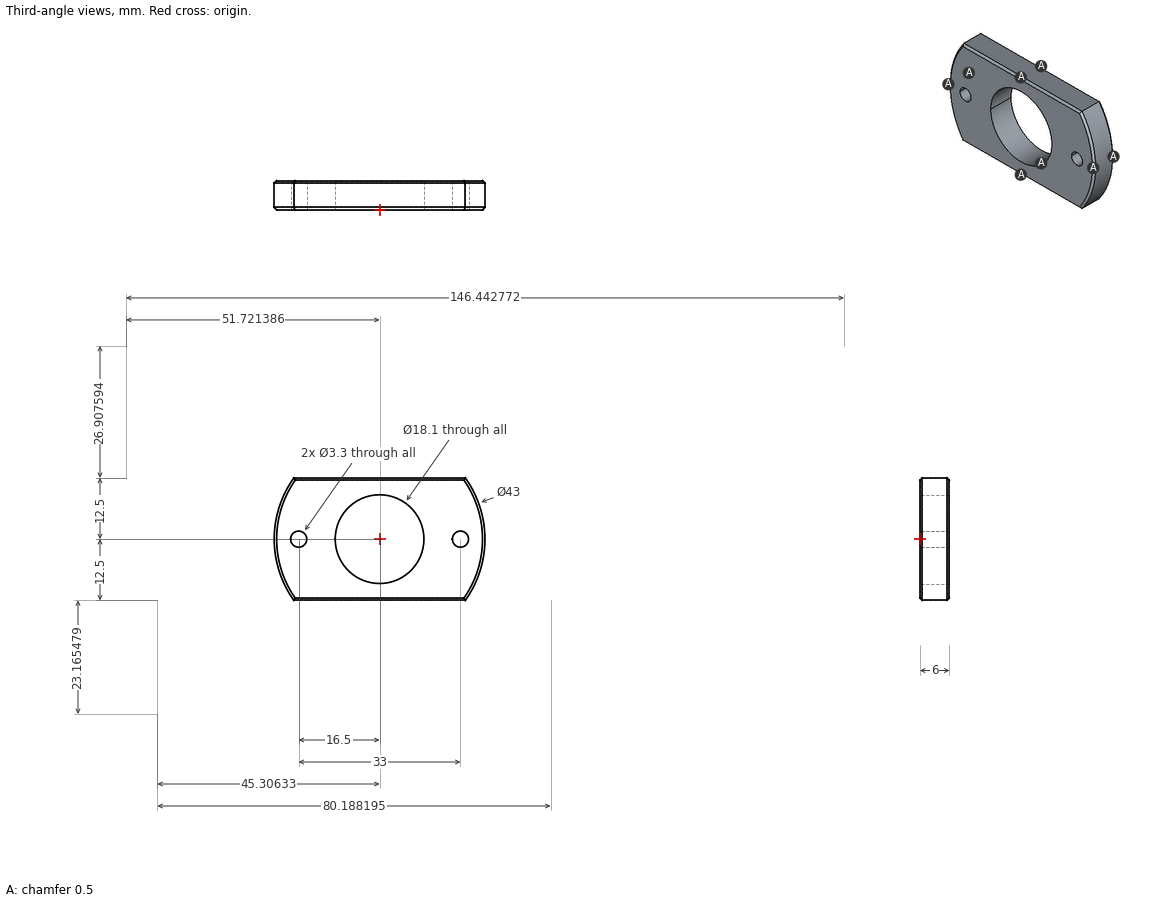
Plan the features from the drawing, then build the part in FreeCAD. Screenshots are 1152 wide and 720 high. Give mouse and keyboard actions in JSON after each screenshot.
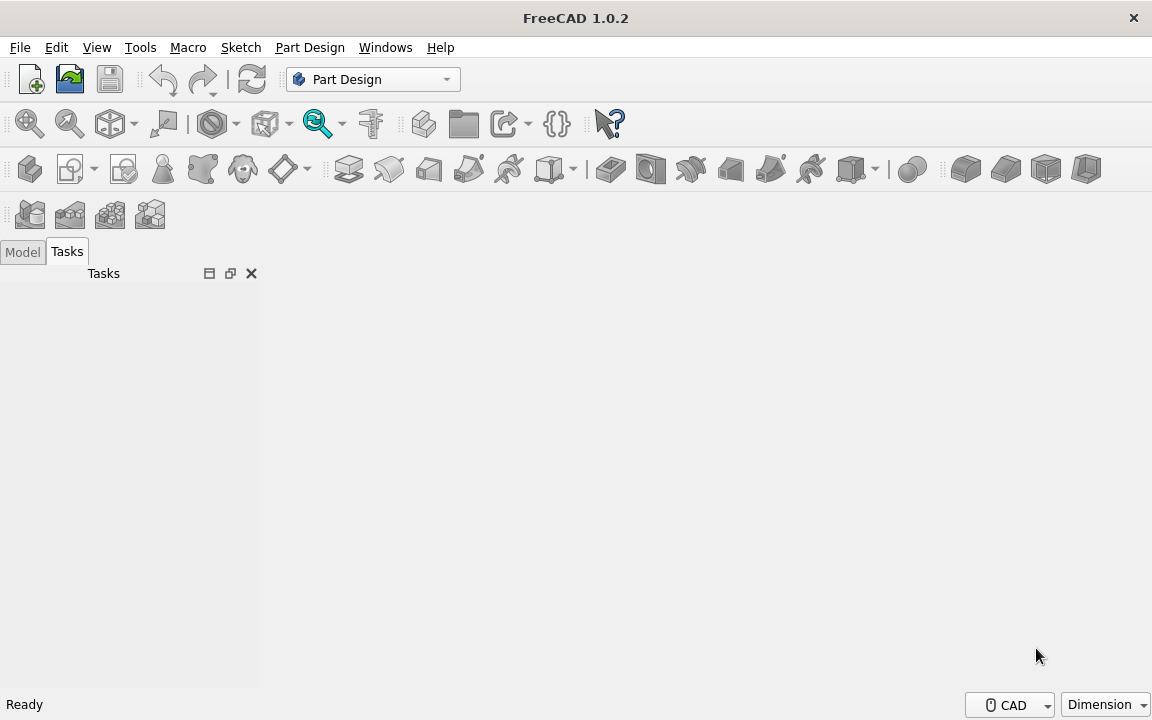
{"action": "left_click", "coordinate": [30, 80]}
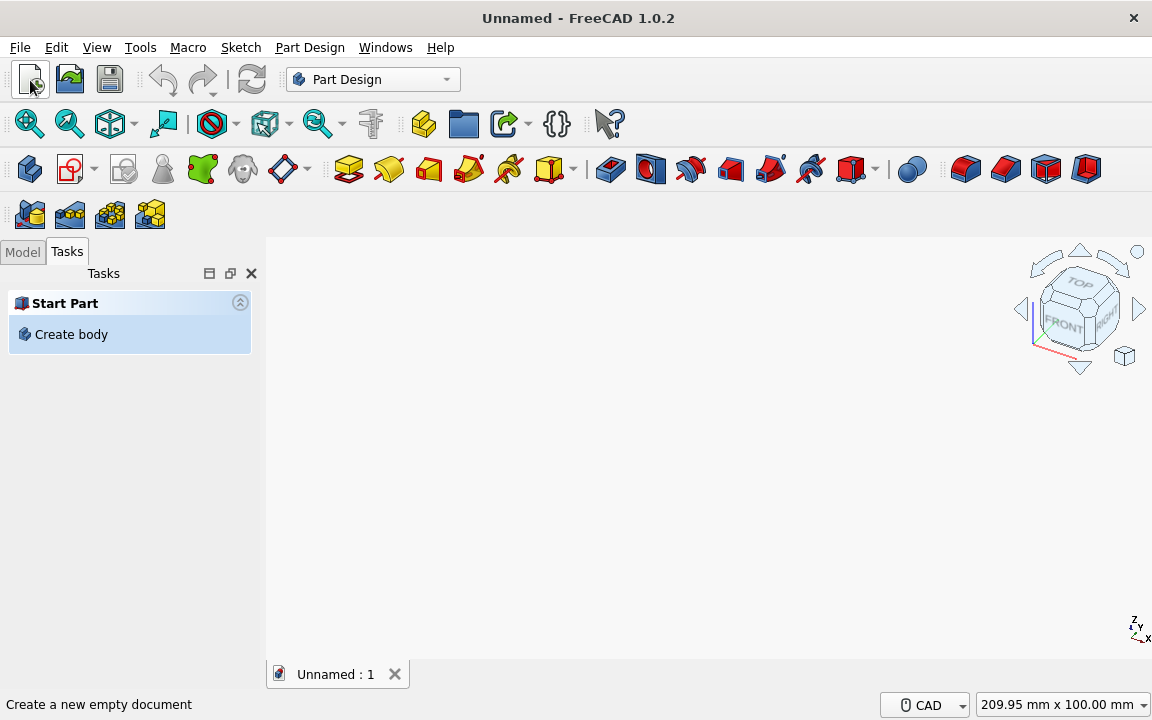
{"action": "left_click", "coordinate": [70, 170]}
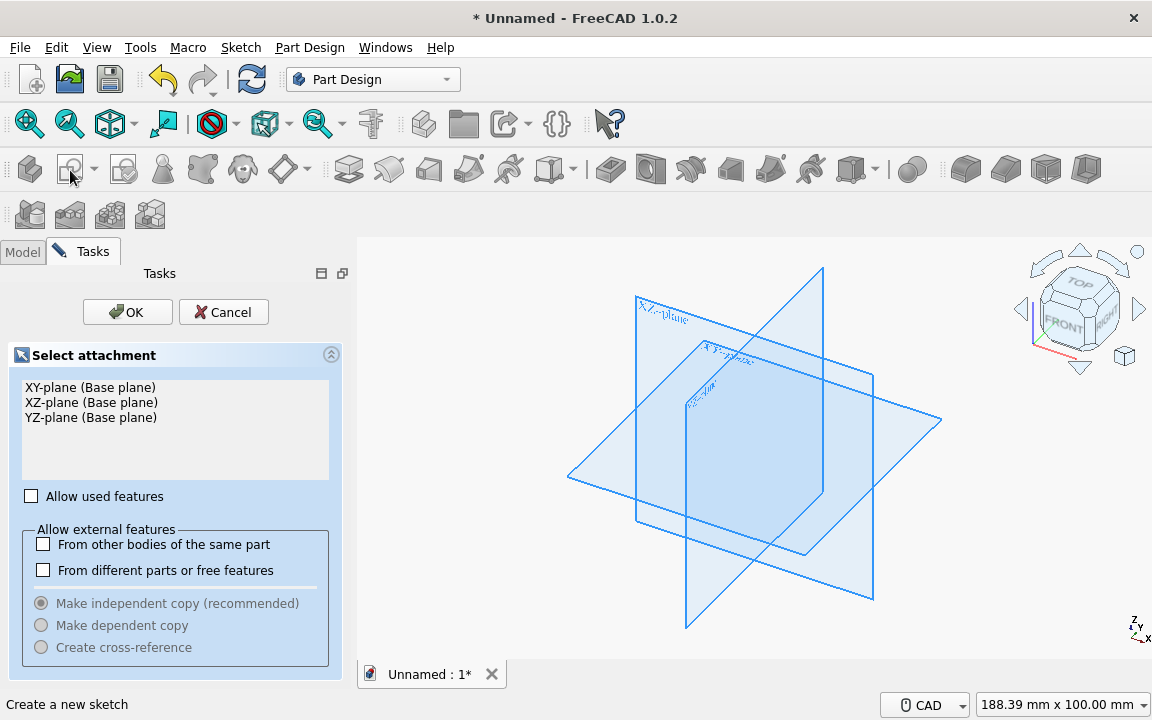
{"action": "left_click", "coordinate": [82, 402]}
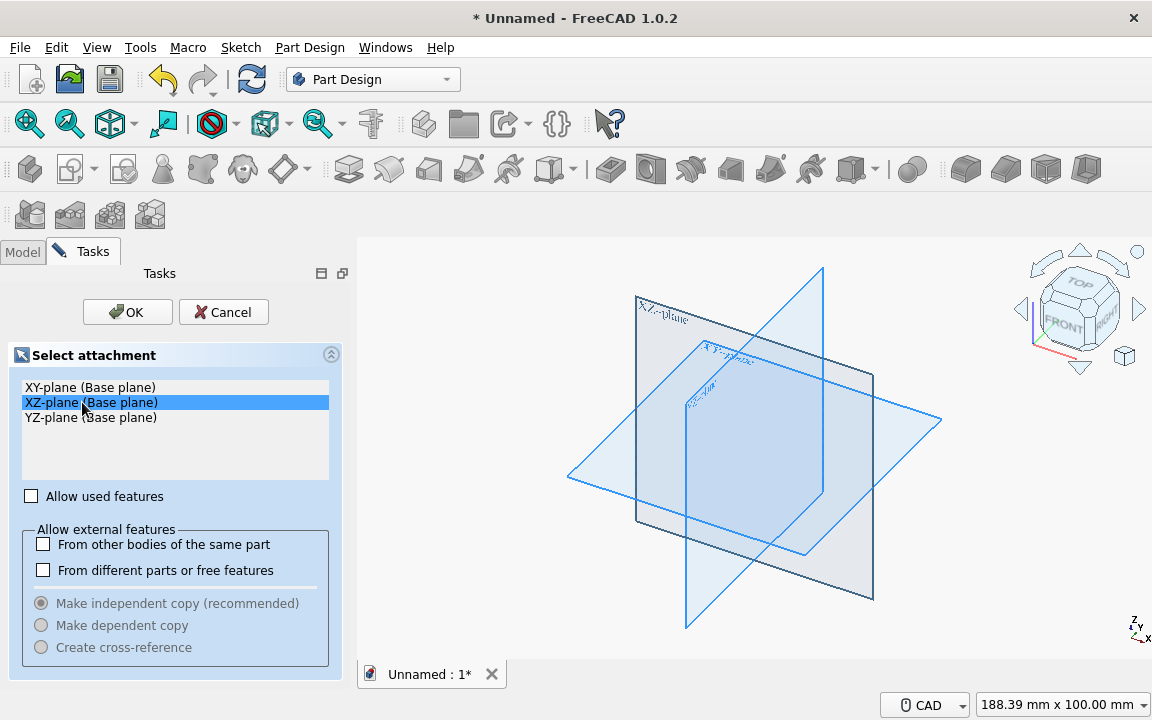
{"action": "left_click", "coordinate": [128, 312]}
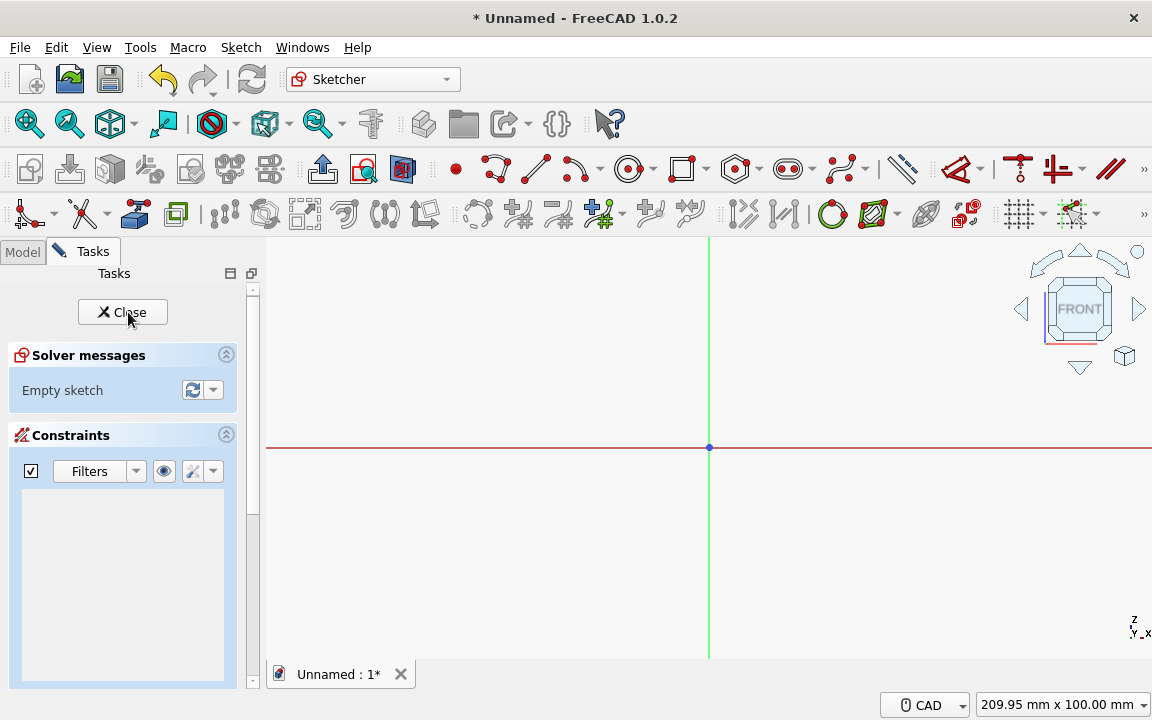
{"action": "scroll", "coordinate": [848, 448], "scroll_direction": "up", "scroll_amount": 2}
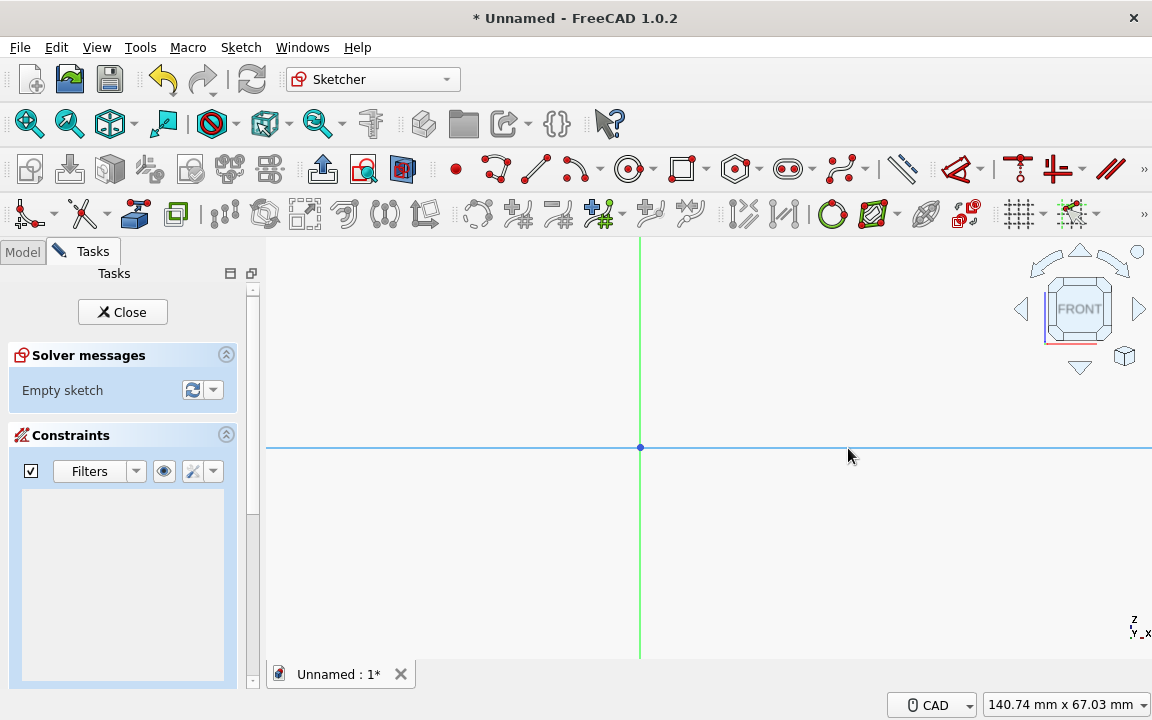
{"action": "left_click", "coordinate": [630, 170]}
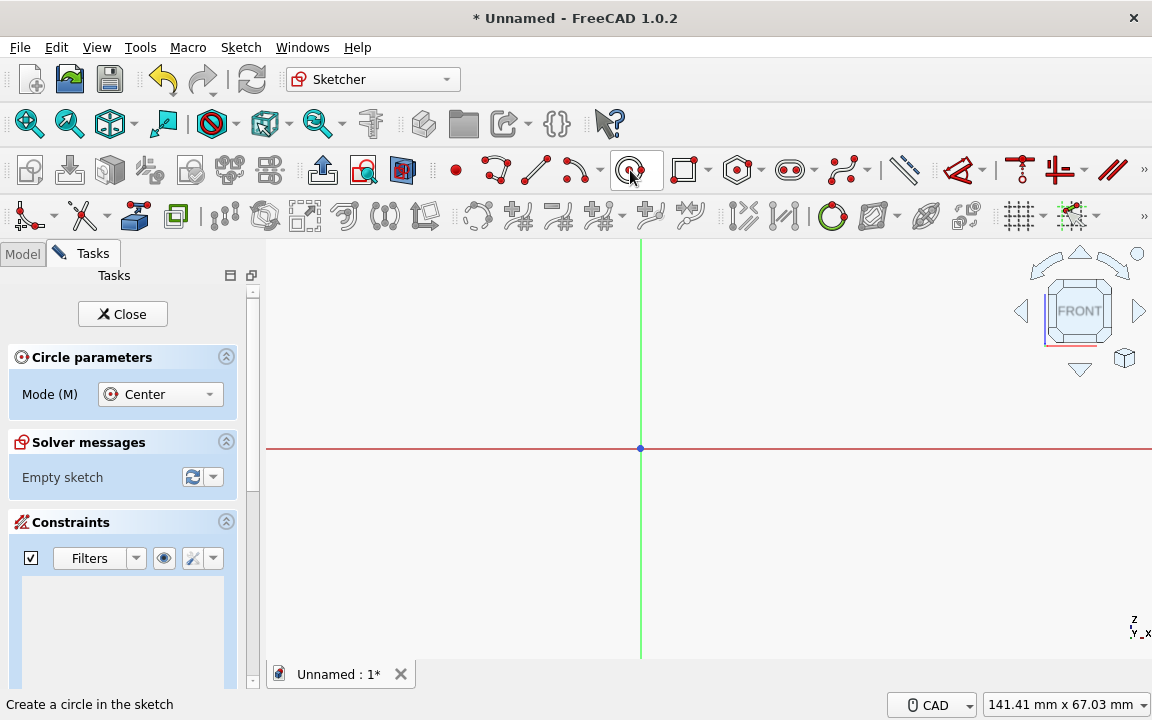
{"action": "left_click", "coordinate": [641, 449]}
{"action": "left_click", "coordinate": [736, 353]}
{"action": "key", "text": "Escape"}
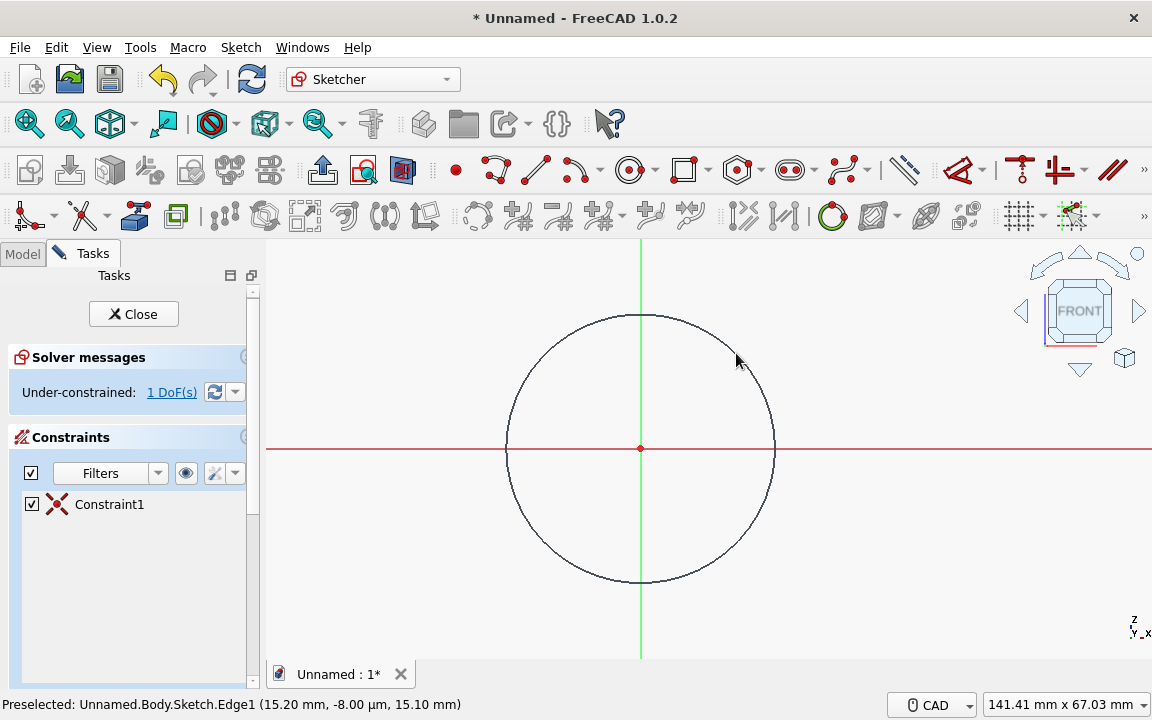
{"action": "left_click", "coordinate": [958, 170]}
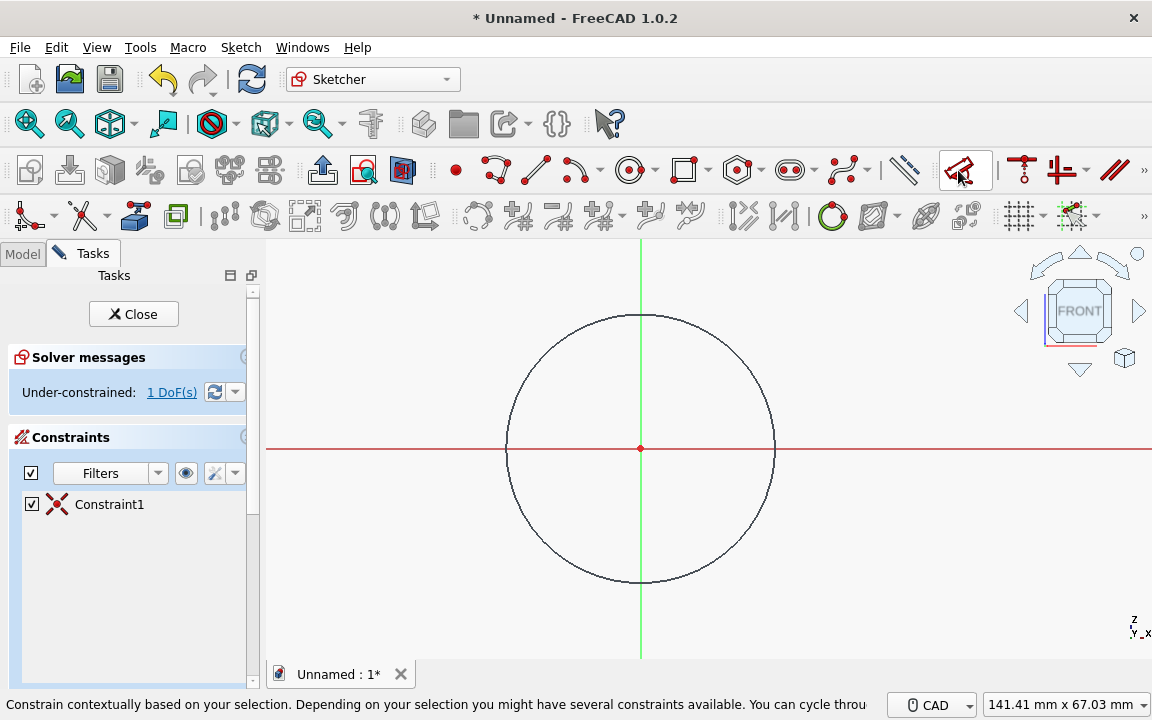
{"action": "left_click", "coordinate": [735, 353]}
{"action": "left_click", "coordinate": [757, 330]}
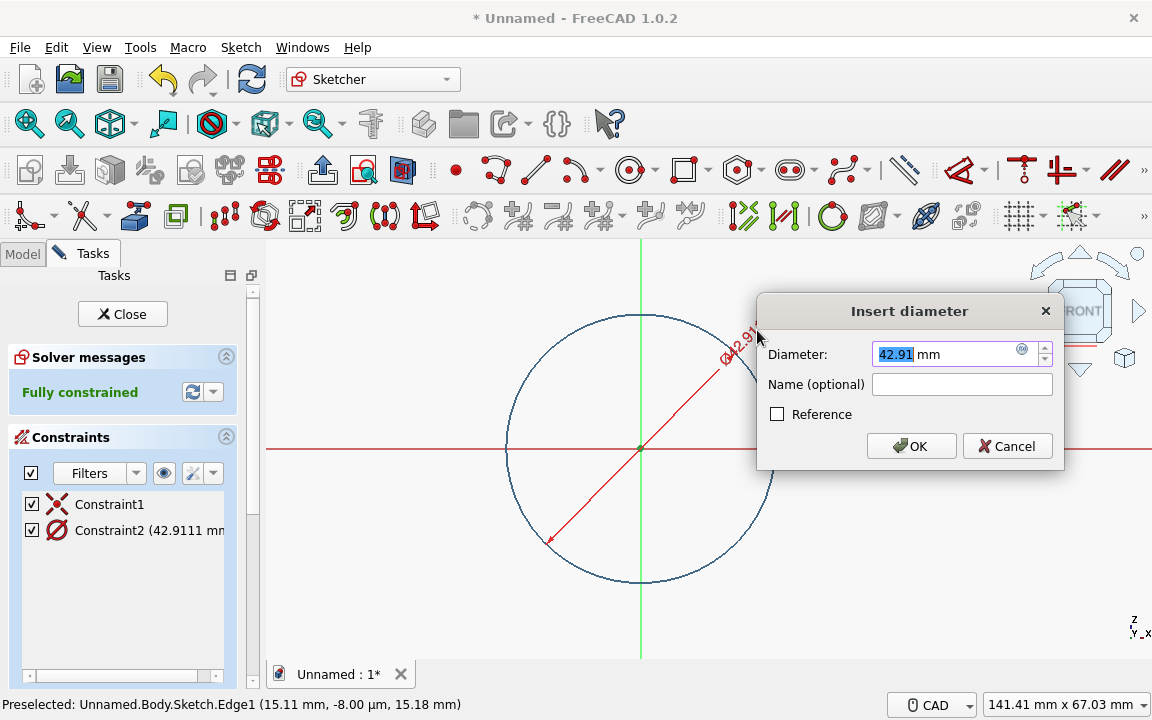
{"action": "type", "text": "43"}
{"action": "key", "text": "Return"}
{"action": "key", "text": "Escape"}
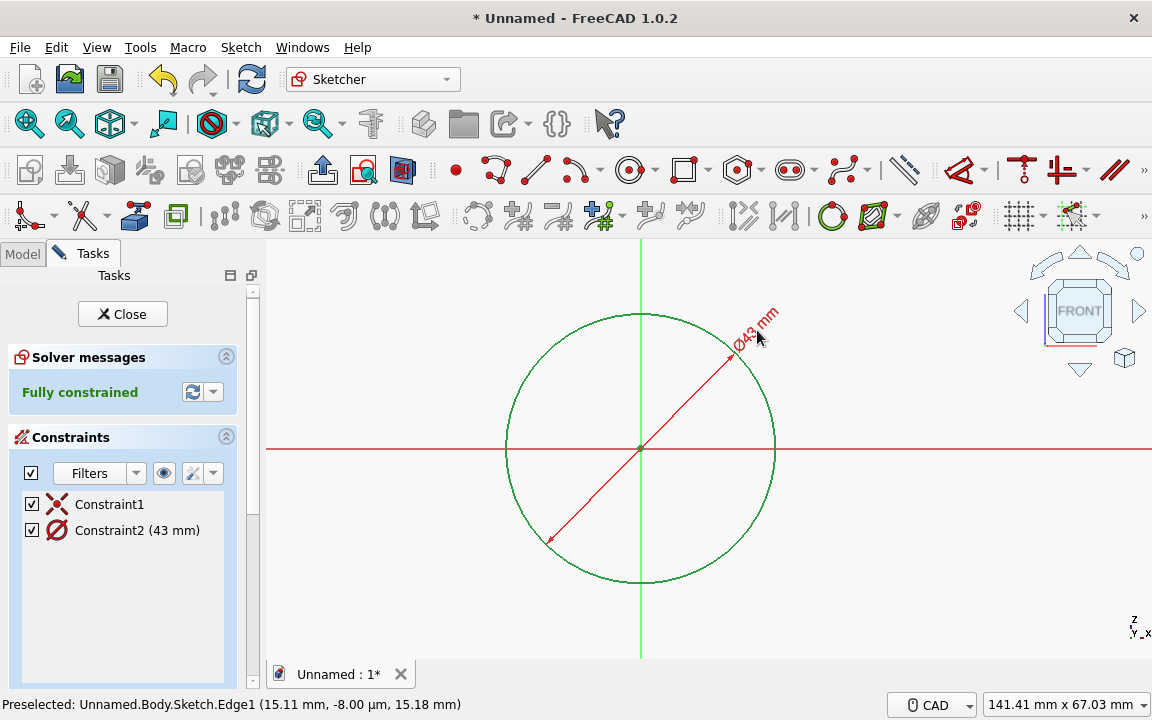
{"action": "left_click", "coordinate": [123, 314]}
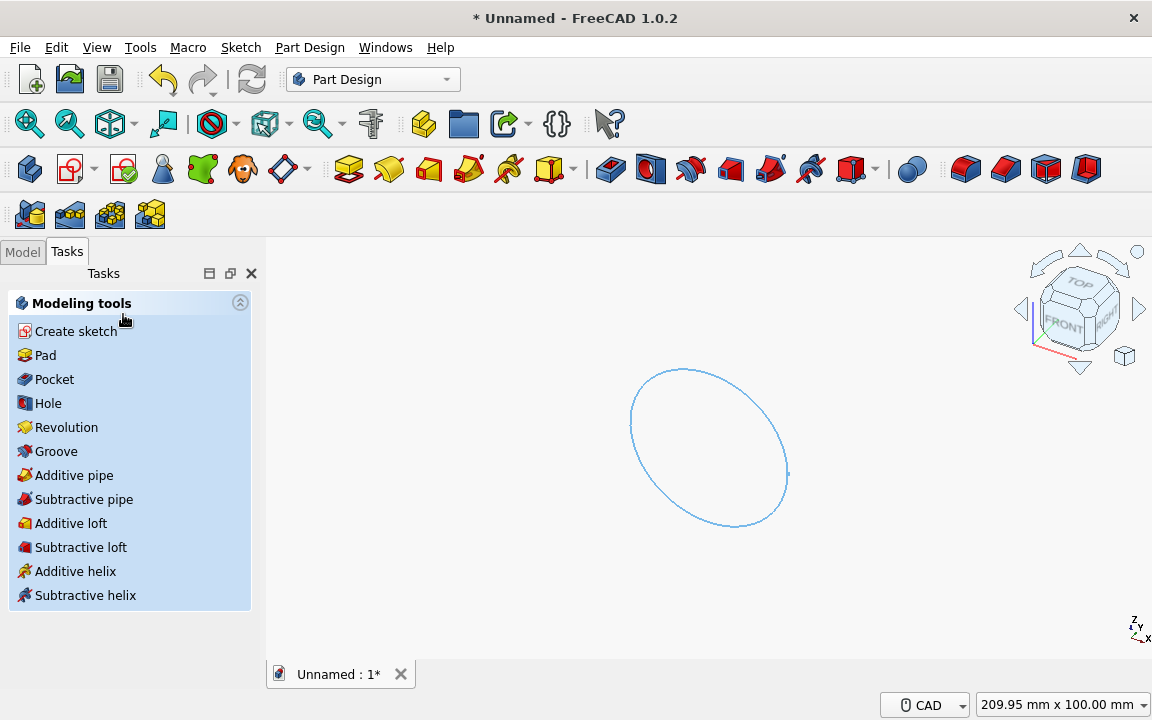
{"action": "left_click", "coordinate": [350, 170]}